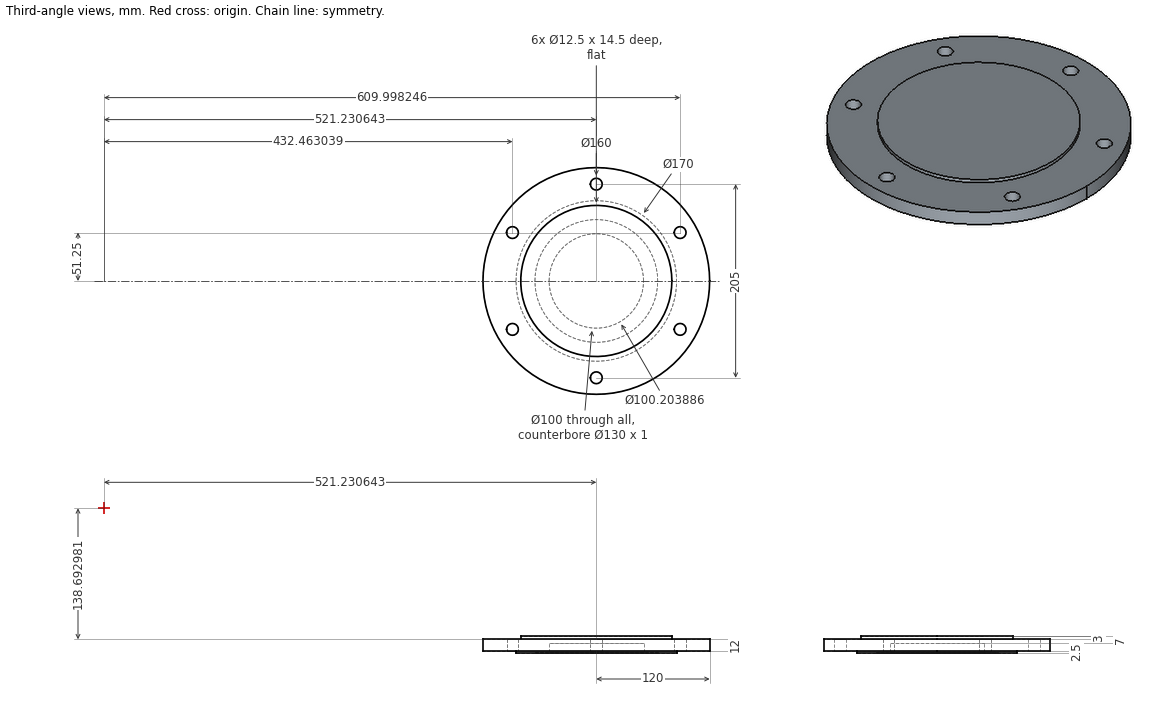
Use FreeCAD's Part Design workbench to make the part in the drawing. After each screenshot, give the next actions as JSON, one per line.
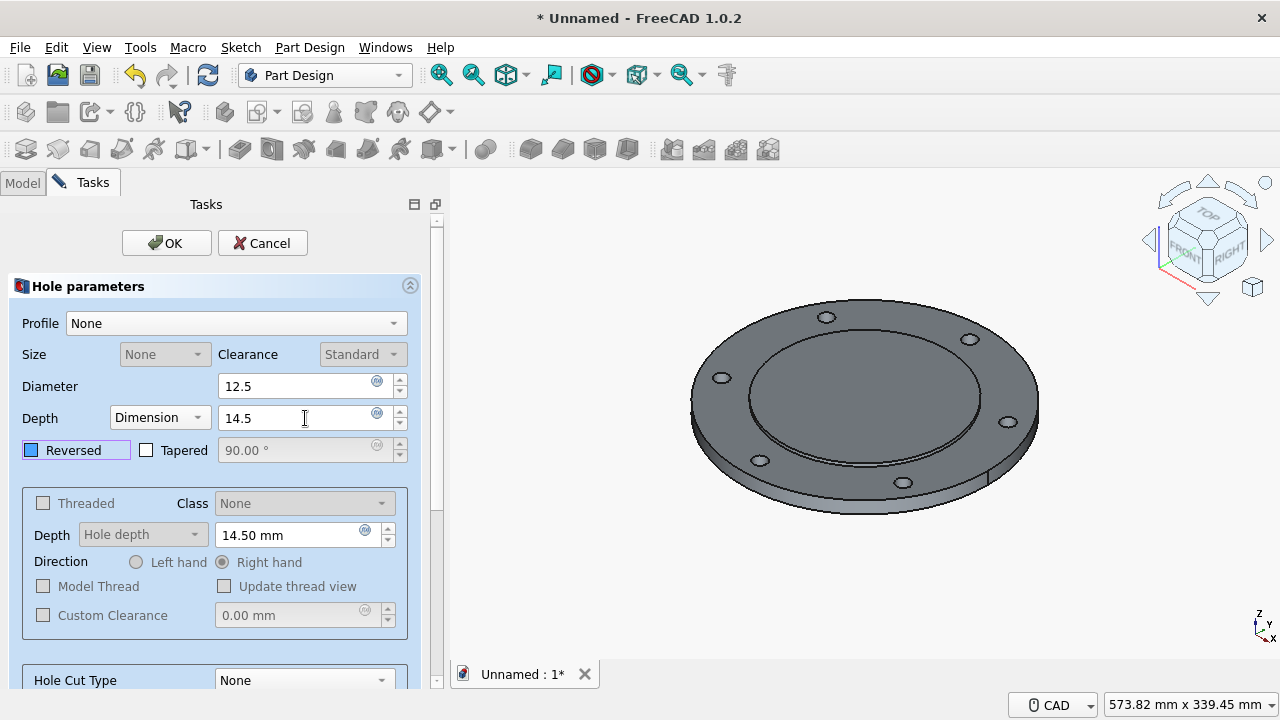
{"action": "scroll", "coordinate": [437, 451], "scroll_direction": "down", "scroll_amount": 5}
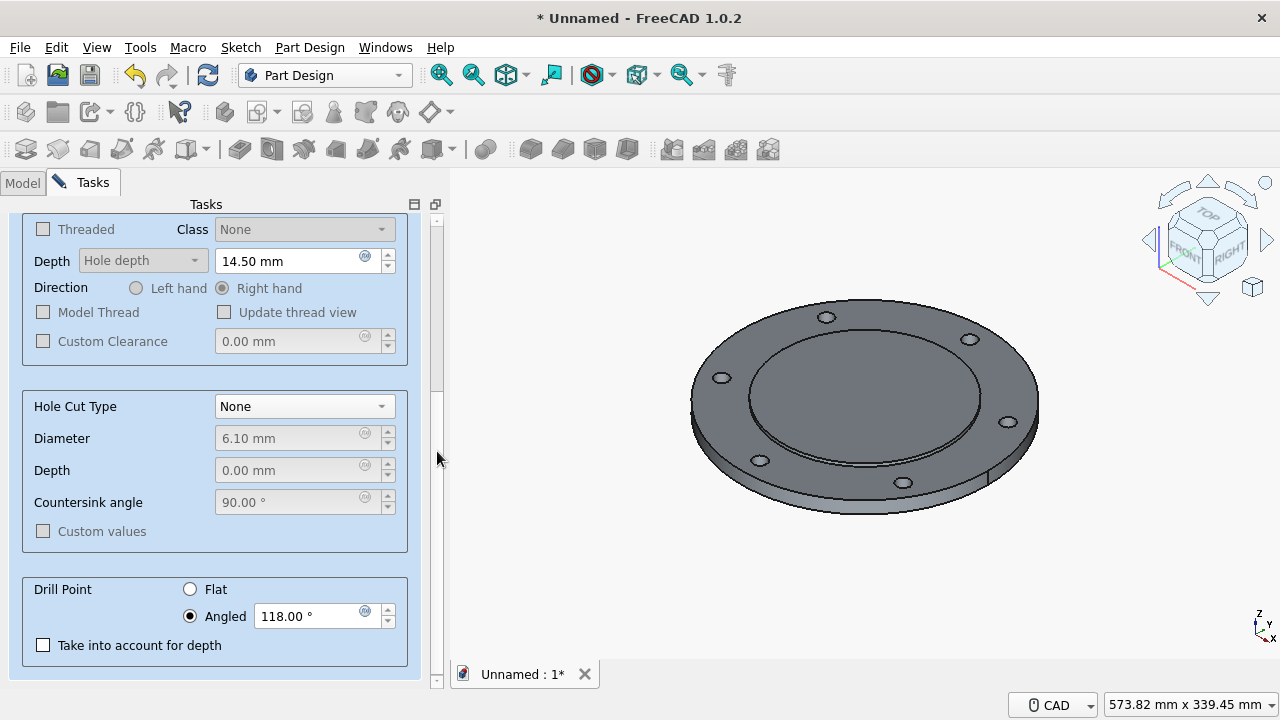
{"action": "left_click", "coordinate": [191, 589]}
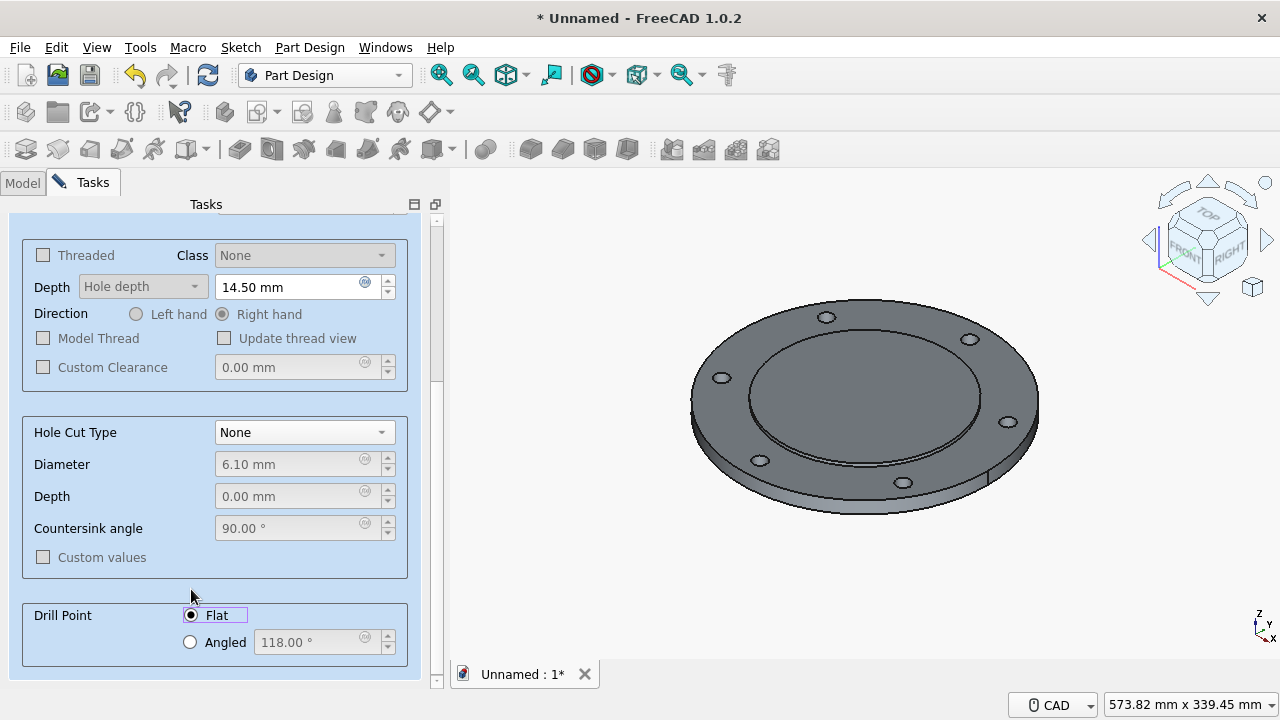
{"action": "scroll", "coordinate": [437, 451], "scroll_direction": "up", "scroll_amount": 5}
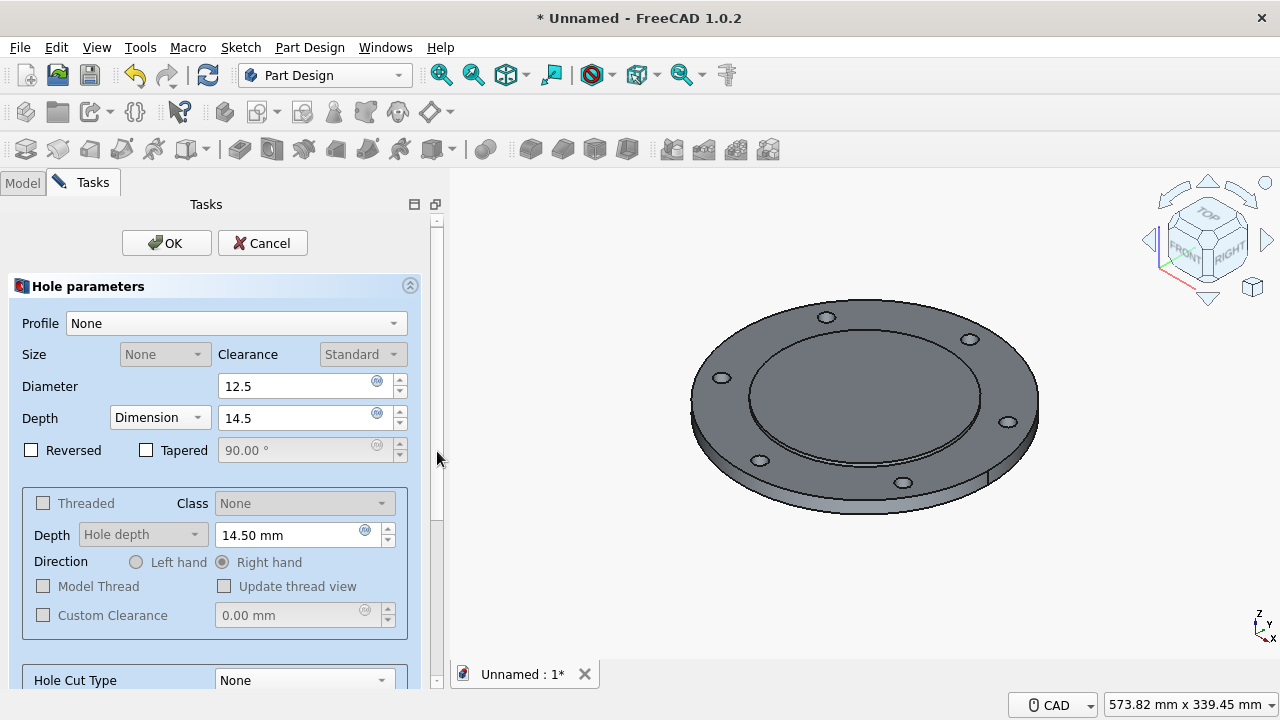
{"action": "left_click", "coordinate": [167, 243]}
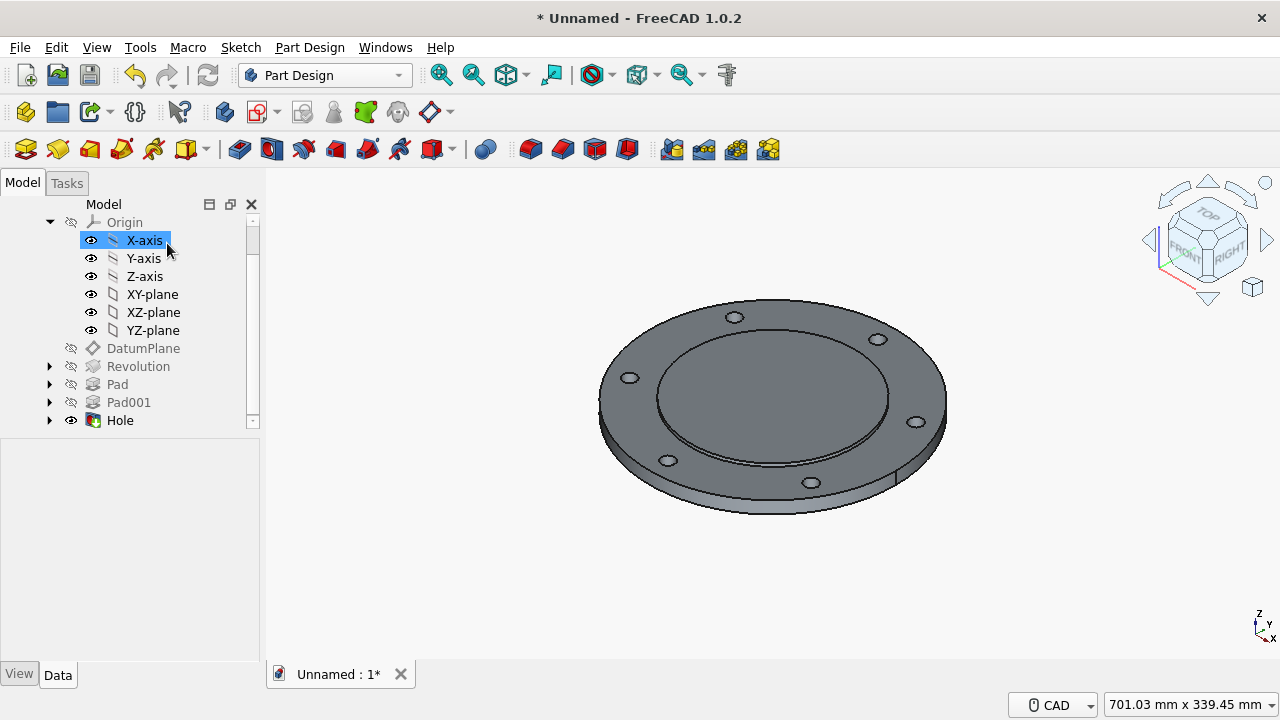
{"action": "key", "text": "5"}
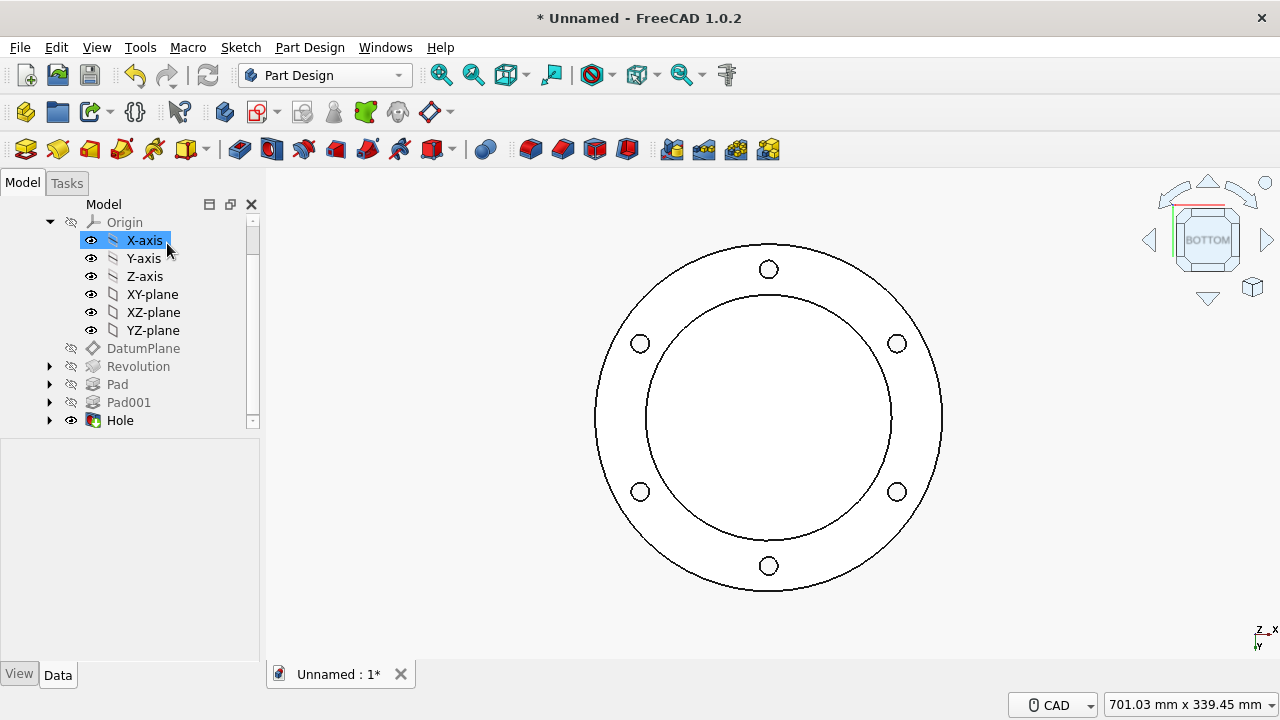
{"action": "left_click", "coordinate": [769, 417]}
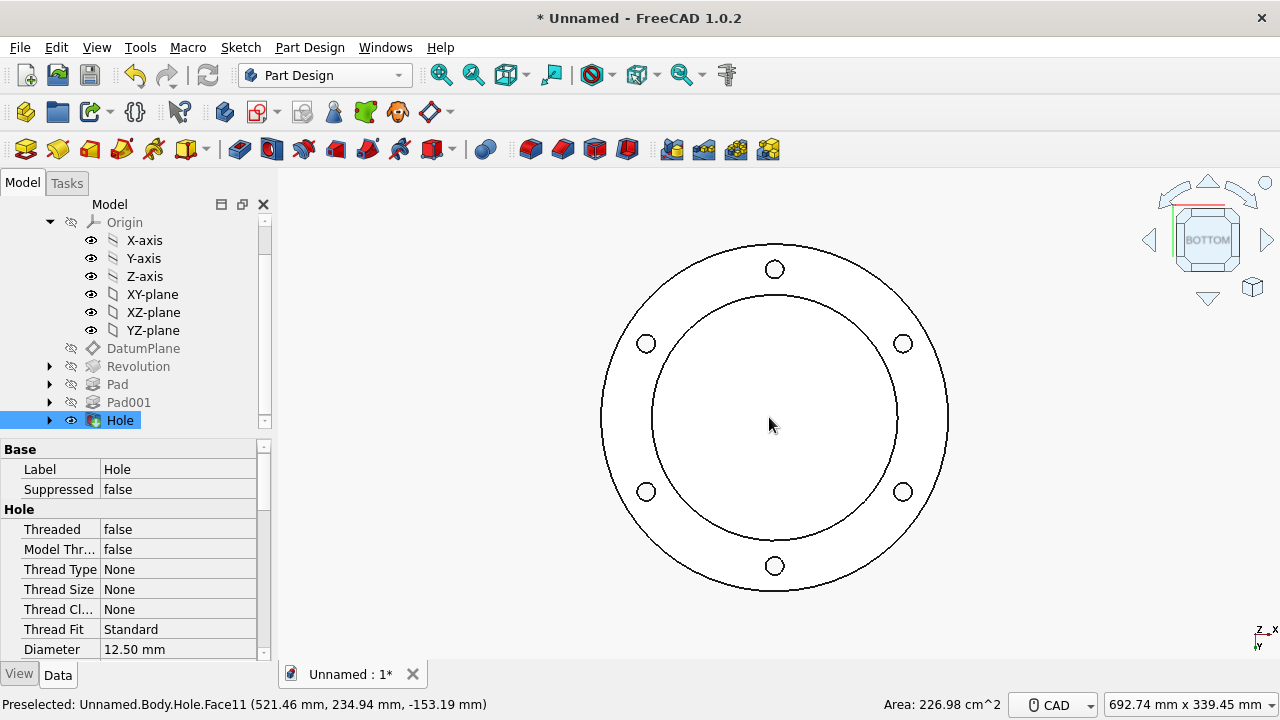
{"action": "left_click", "coordinate": [258, 112]}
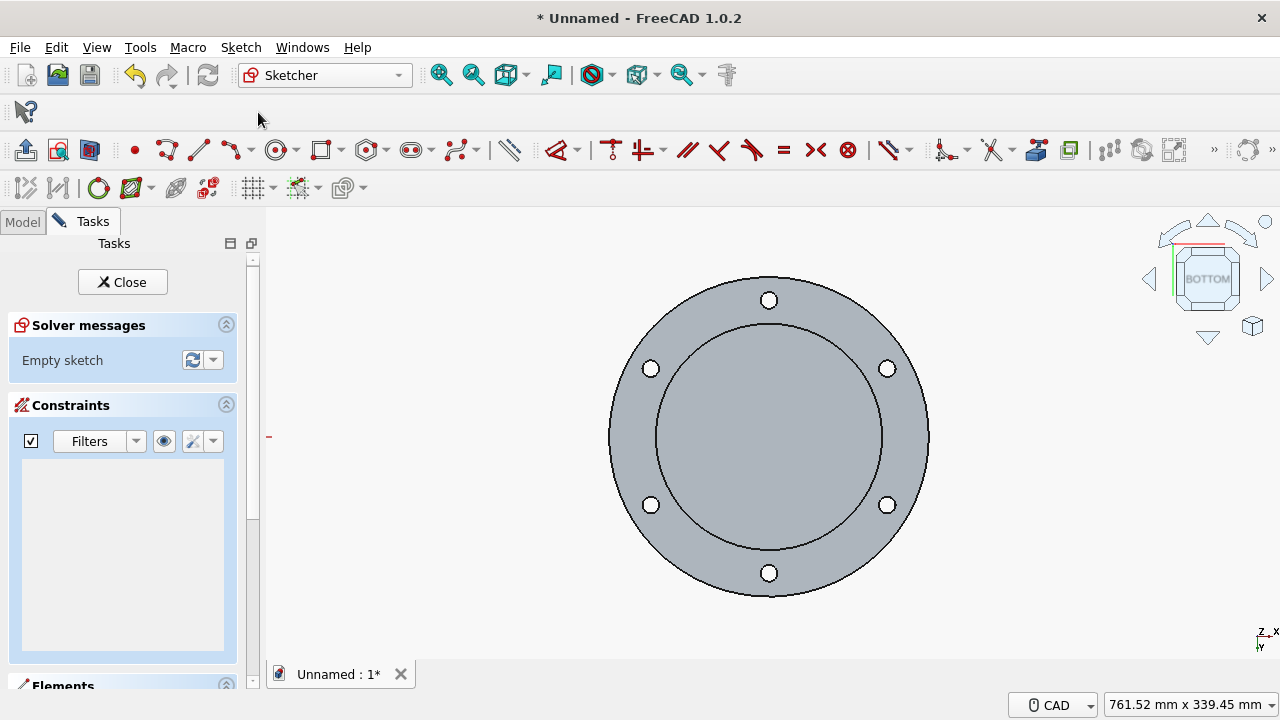
{"action": "scroll", "coordinate": [822, 440], "scroll_direction": "up", "scroll_amount": 4}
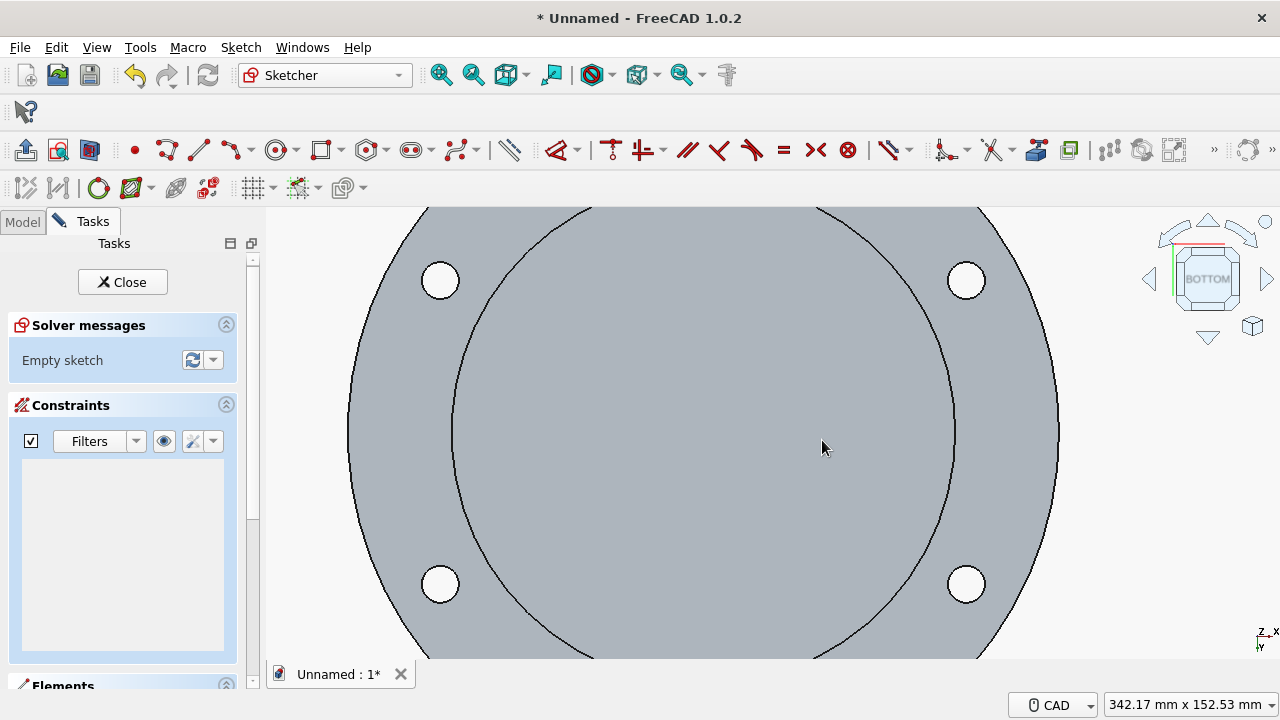
{"action": "key", "text": "g c"}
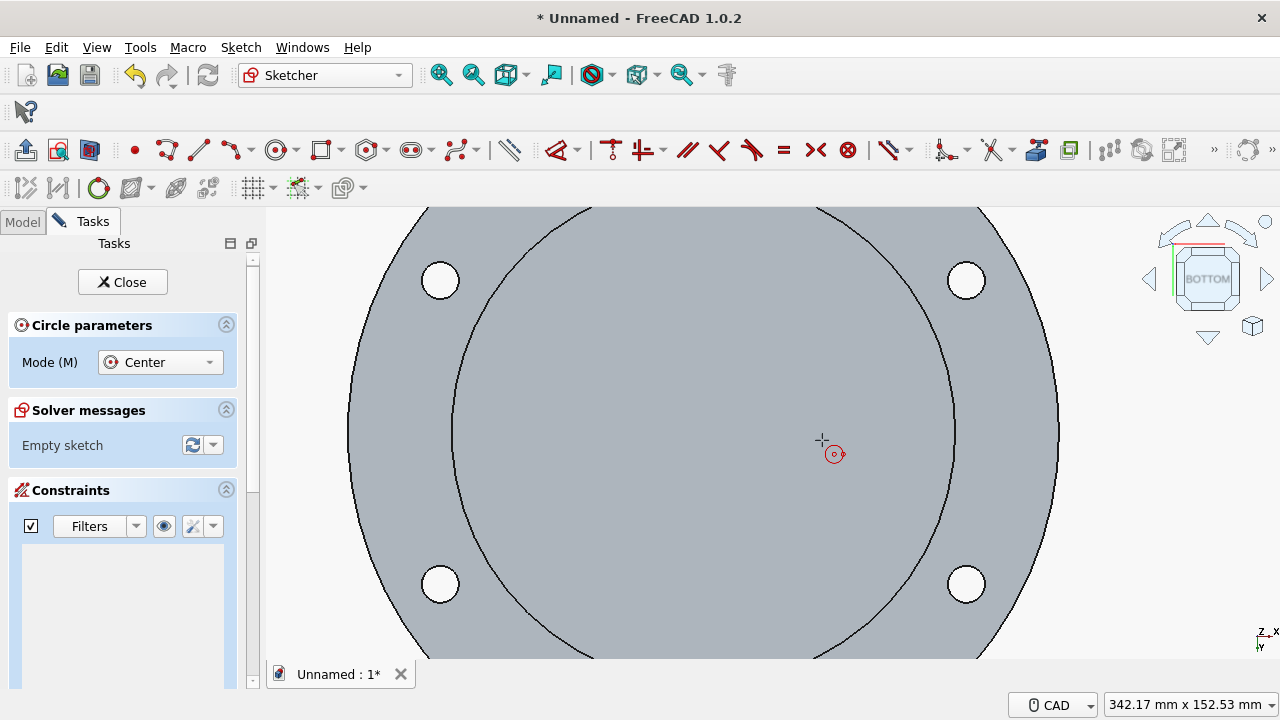
{"action": "left_click", "coordinate": [703, 432]}
{"action": "mouse_move", "coordinate": [808, 328]}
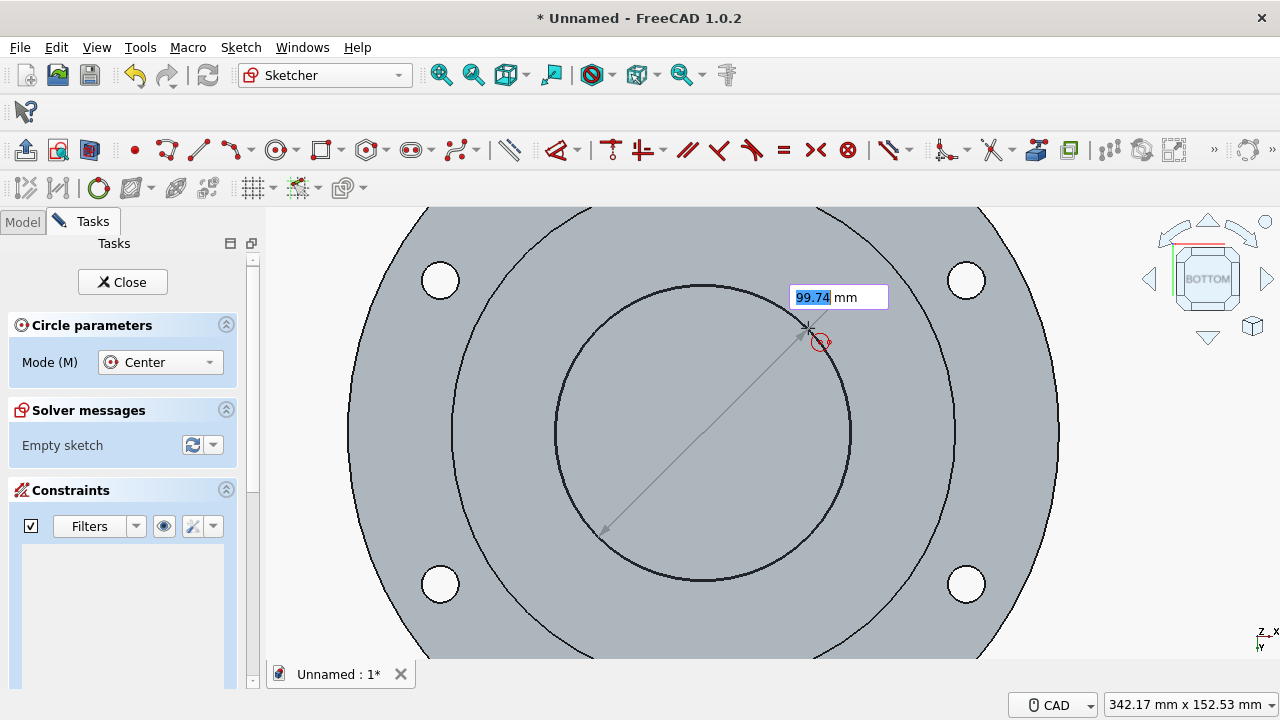
{"action": "type", "text": "100"}
{"action": "key", "text": "Return"}
{"action": "key", "text": "Escape"}